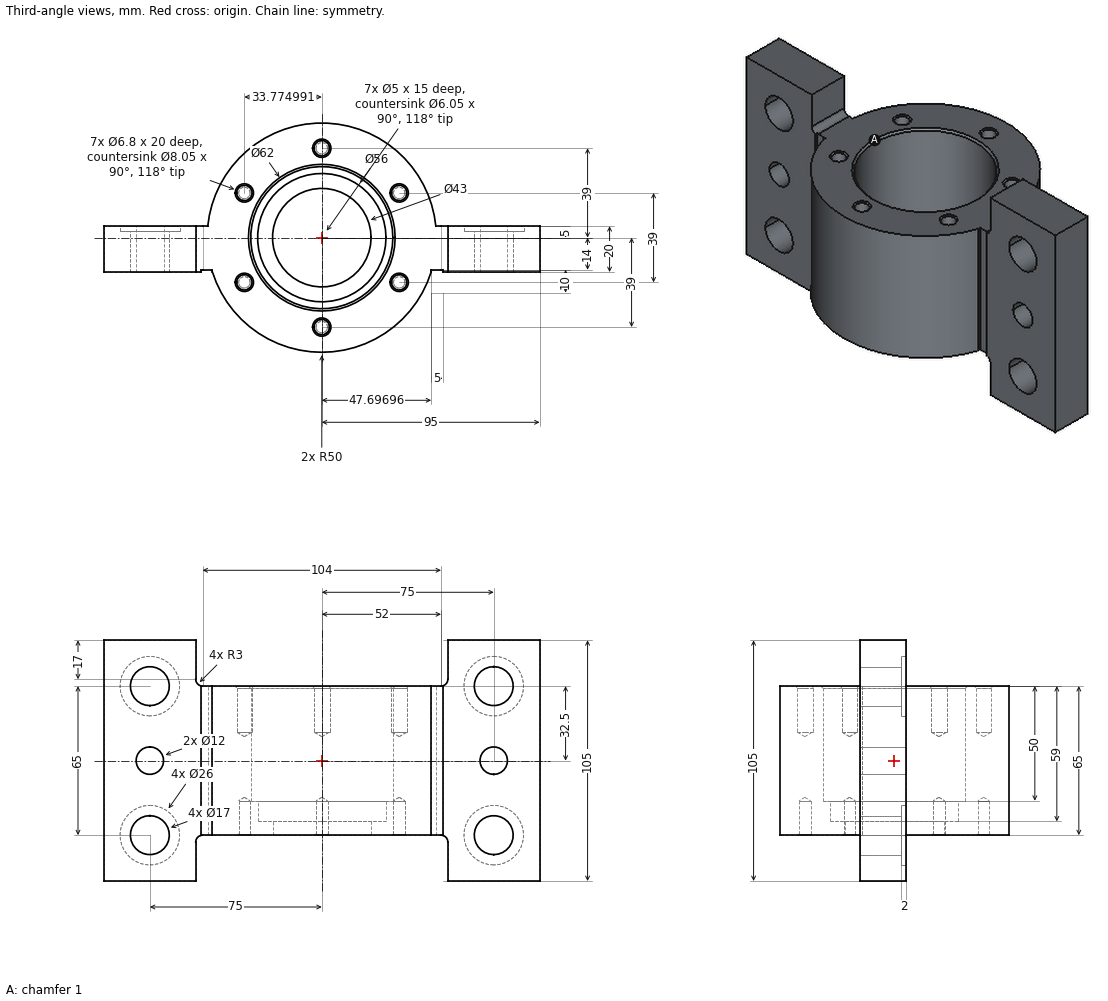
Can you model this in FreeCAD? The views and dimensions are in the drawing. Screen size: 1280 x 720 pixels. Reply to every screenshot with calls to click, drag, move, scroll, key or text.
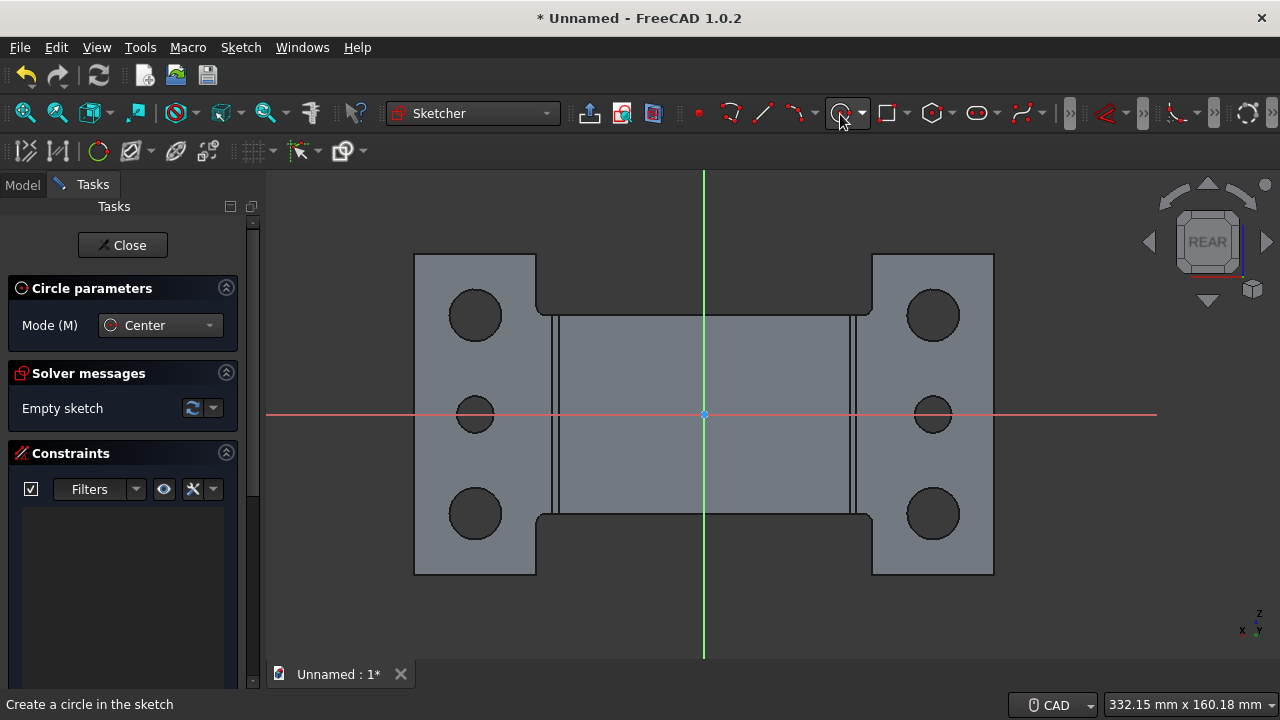
click(933, 514)
click(961, 486)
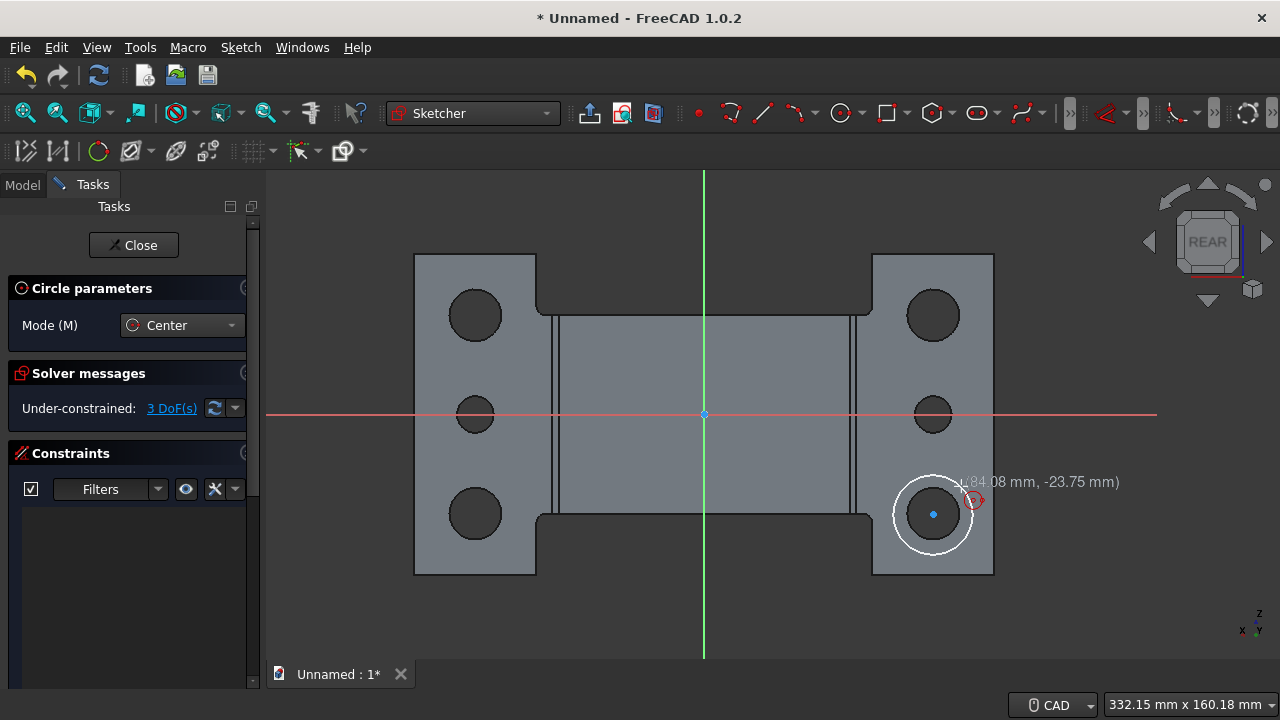
click(475, 514)
click(503, 486)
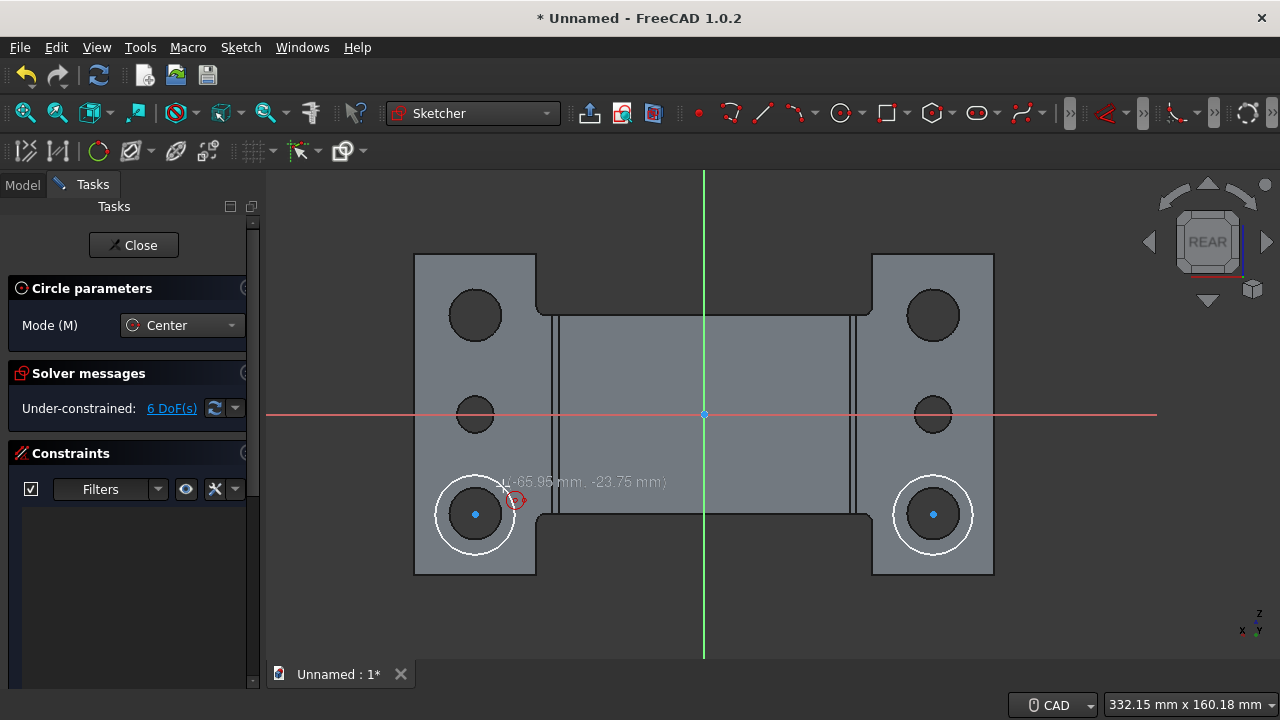
click(475, 315)
click(503, 287)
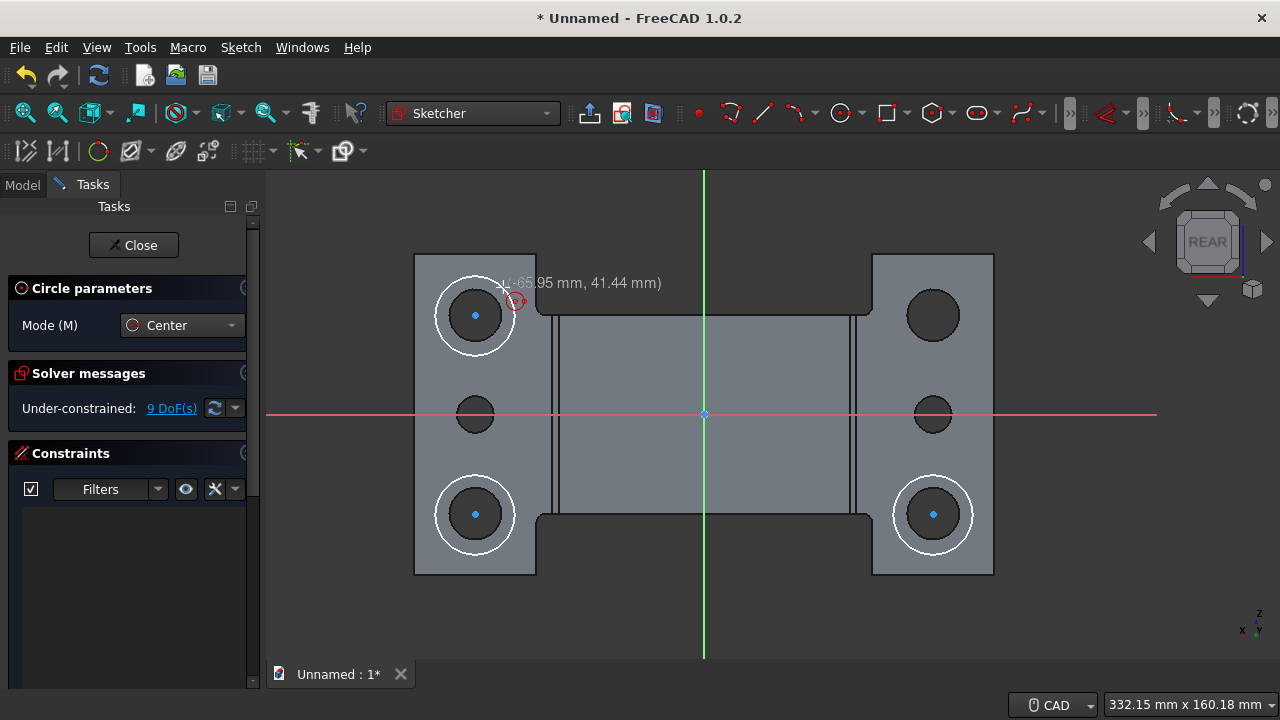
click(933, 315)
click(961, 287)
key(Escape)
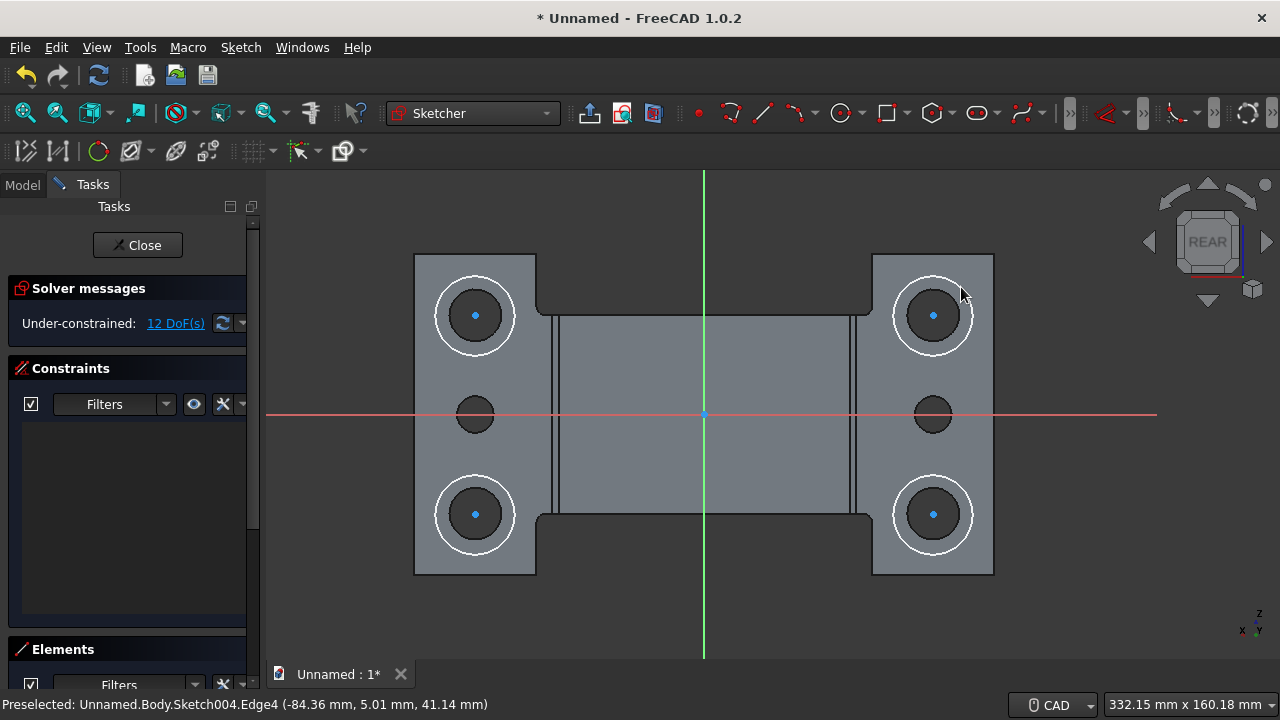
click(961, 487)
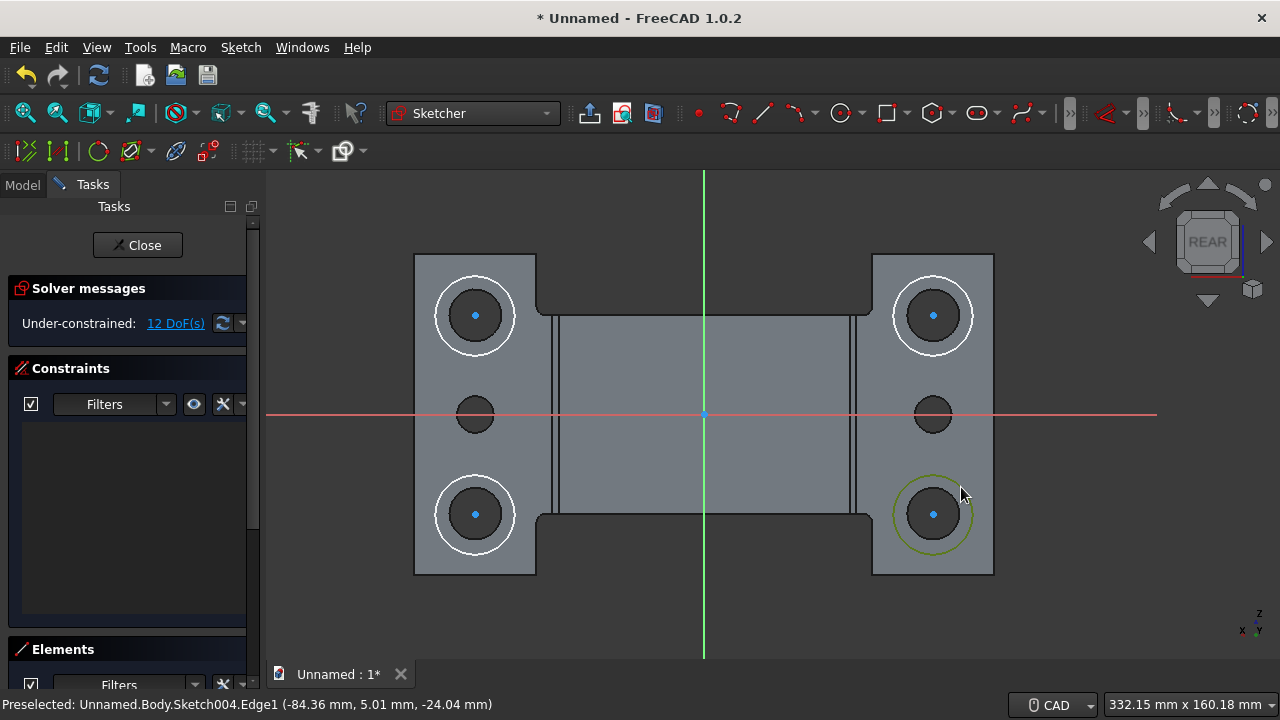
click(503, 487)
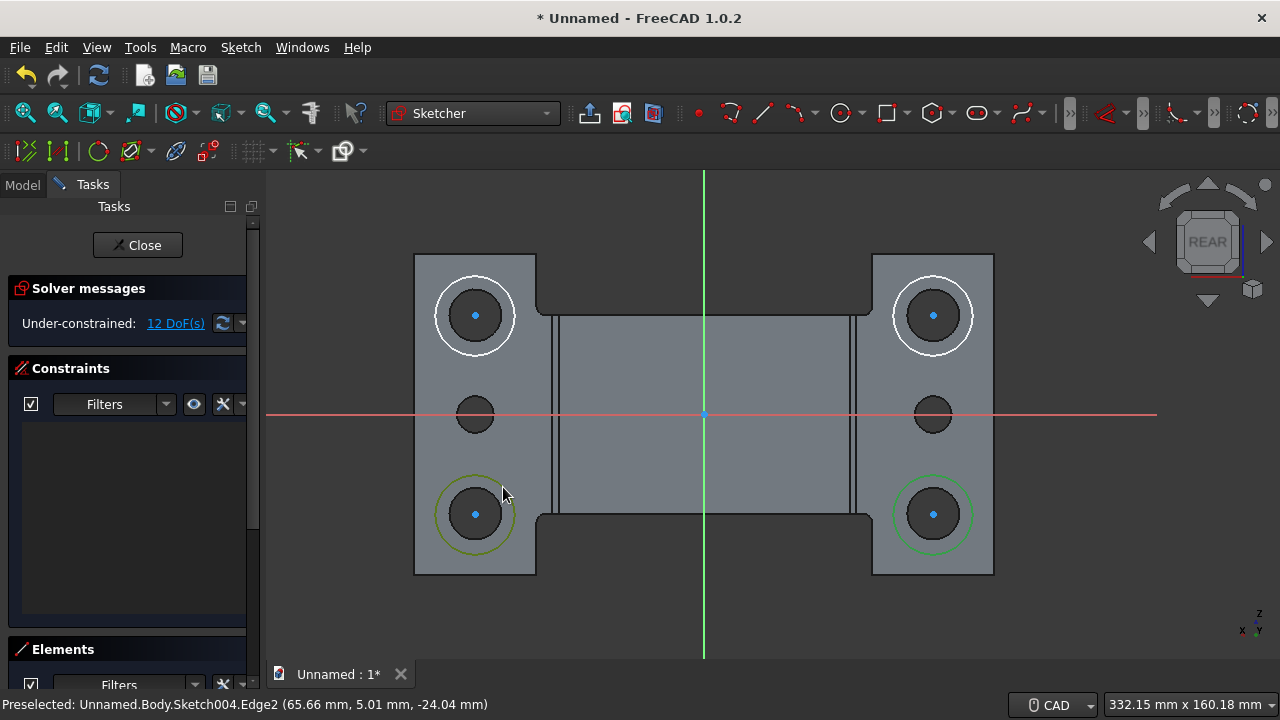
click(503, 288)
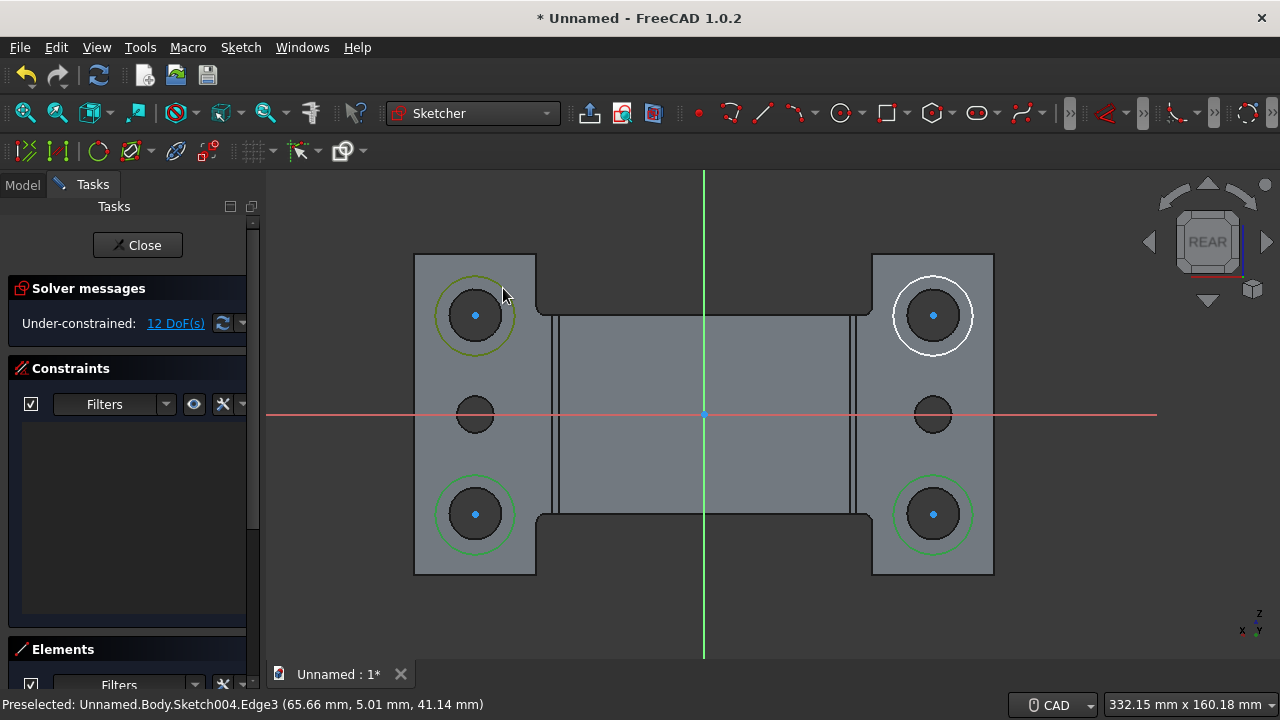
click(961, 288)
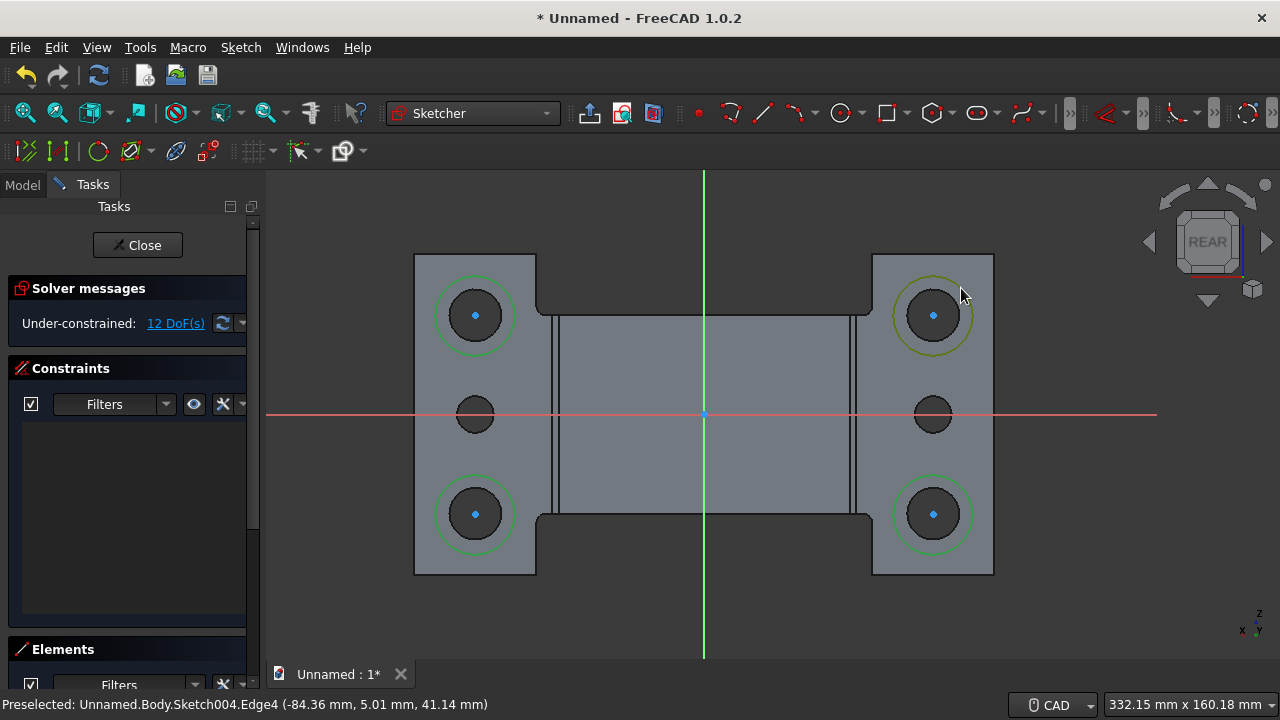
key(e)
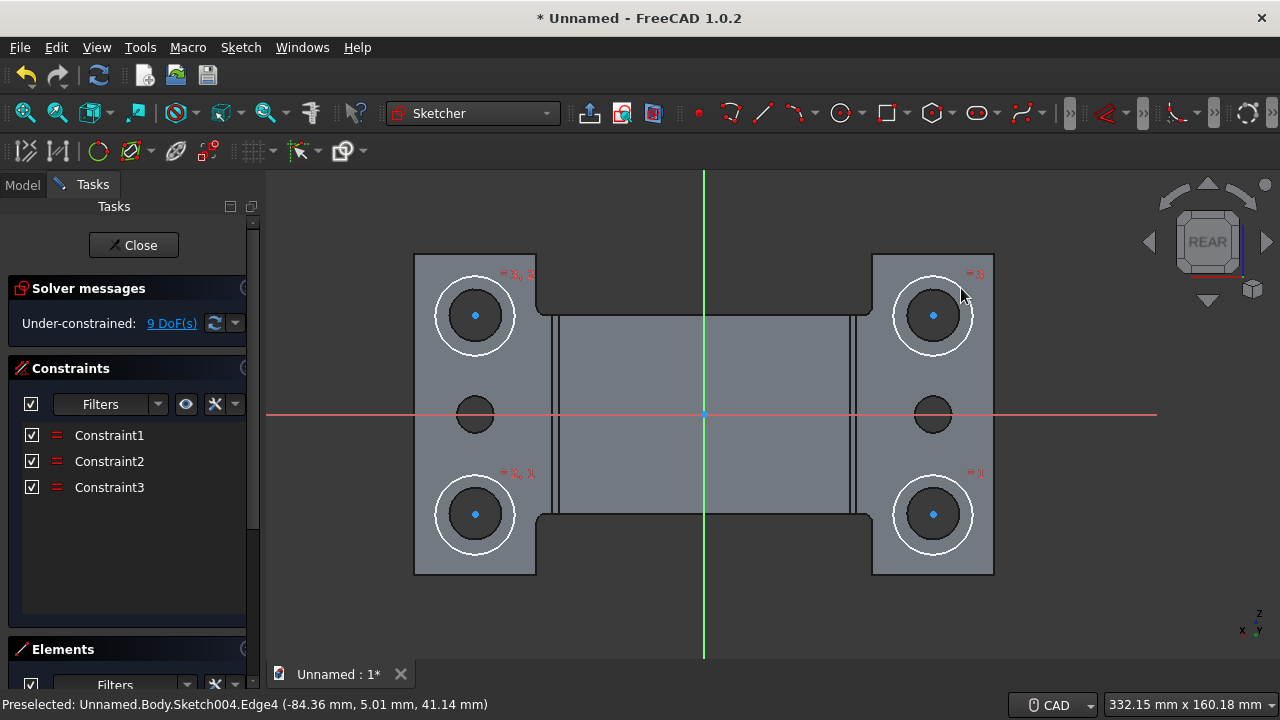
click(933, 515)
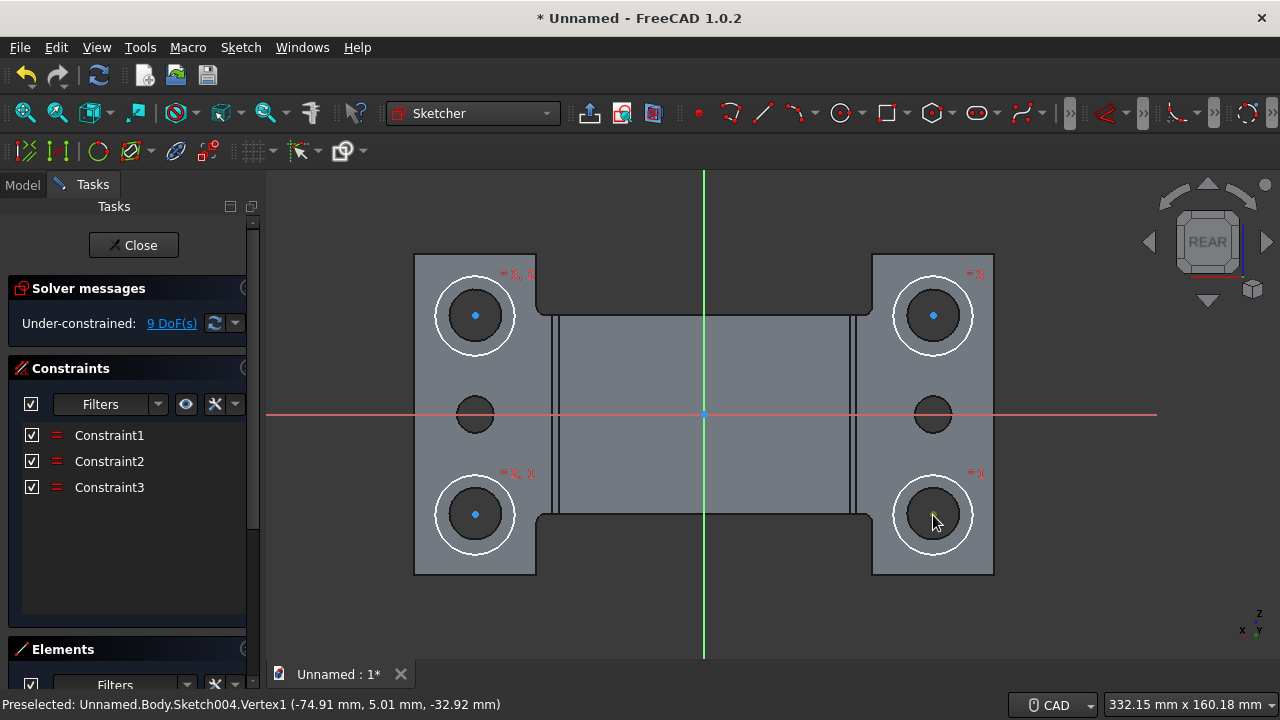
click(475, 515)